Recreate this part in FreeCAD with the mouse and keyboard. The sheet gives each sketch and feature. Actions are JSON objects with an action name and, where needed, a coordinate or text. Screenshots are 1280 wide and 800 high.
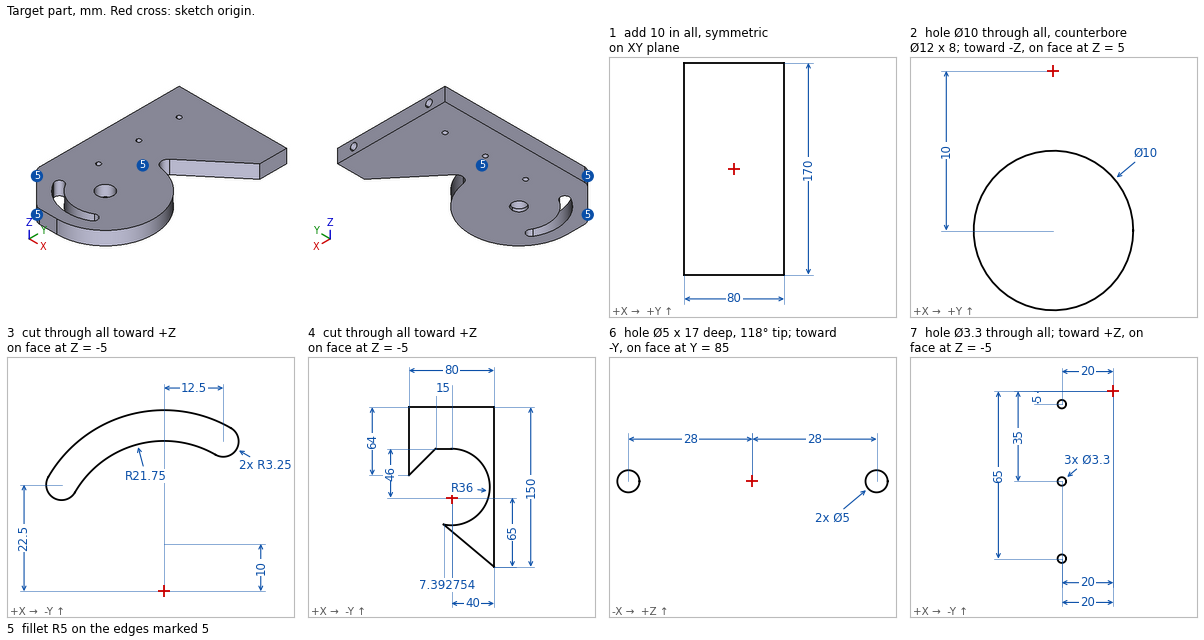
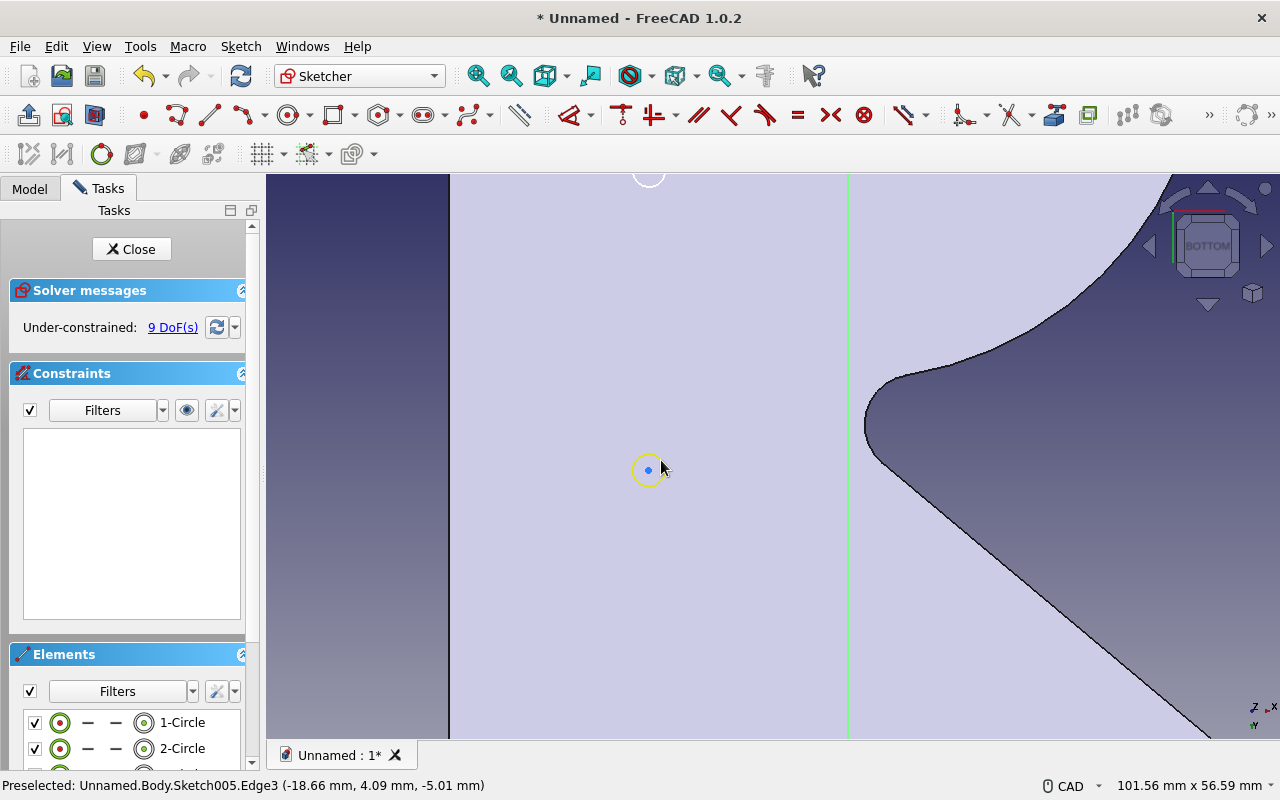
{"action": "left_click", "coordinate": [660, 459]}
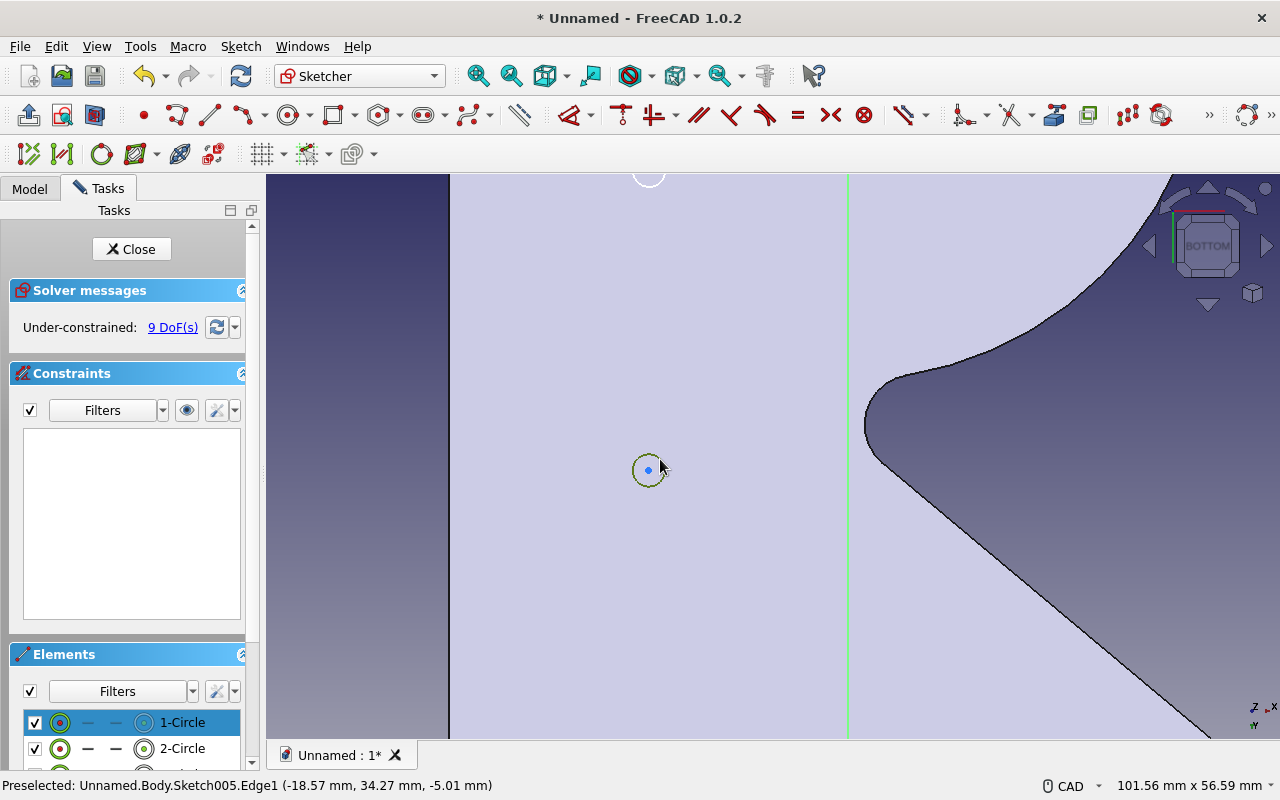
{"action": "scroll", "coordinate": [661, 460], "scroll_direction": "down", "scroll_amount": 3}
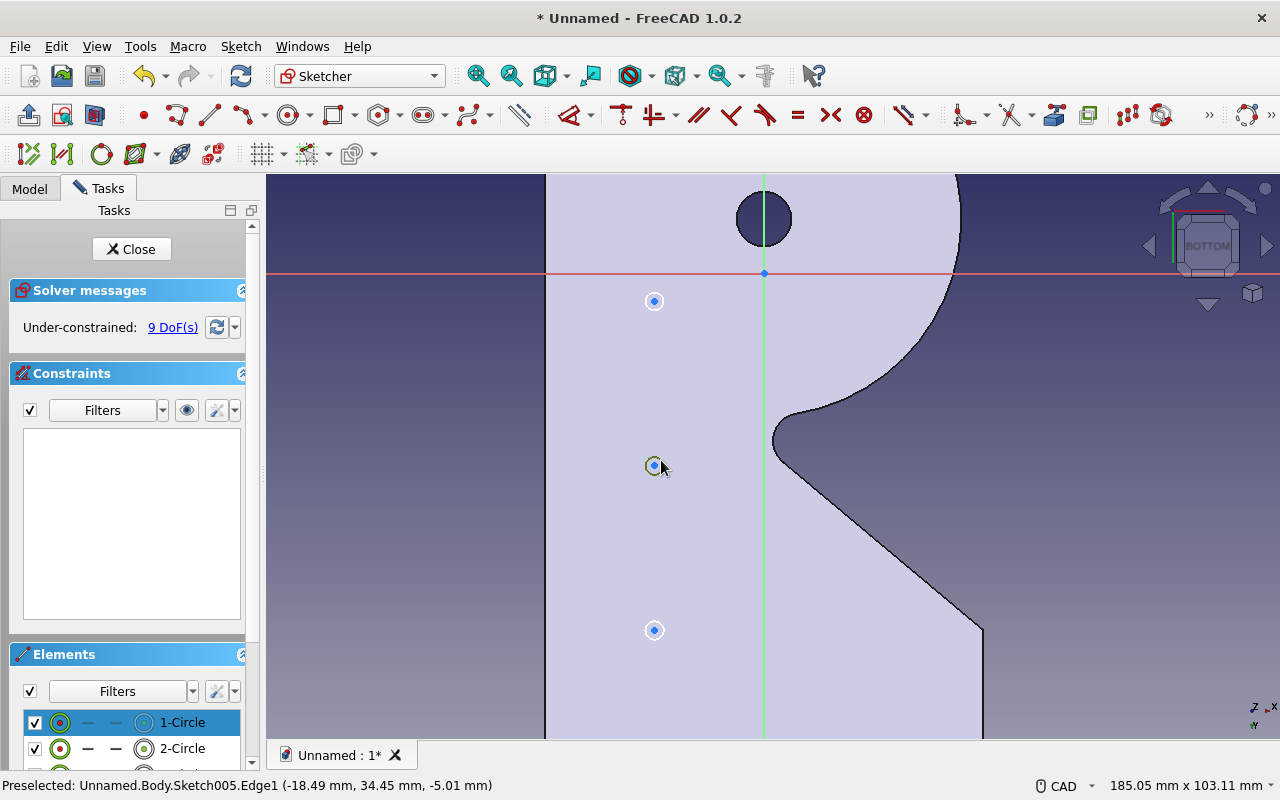
{"action": "scroll", "coordinate": [661, 624], "scroll_direction": "up", "scroll_amount": 3}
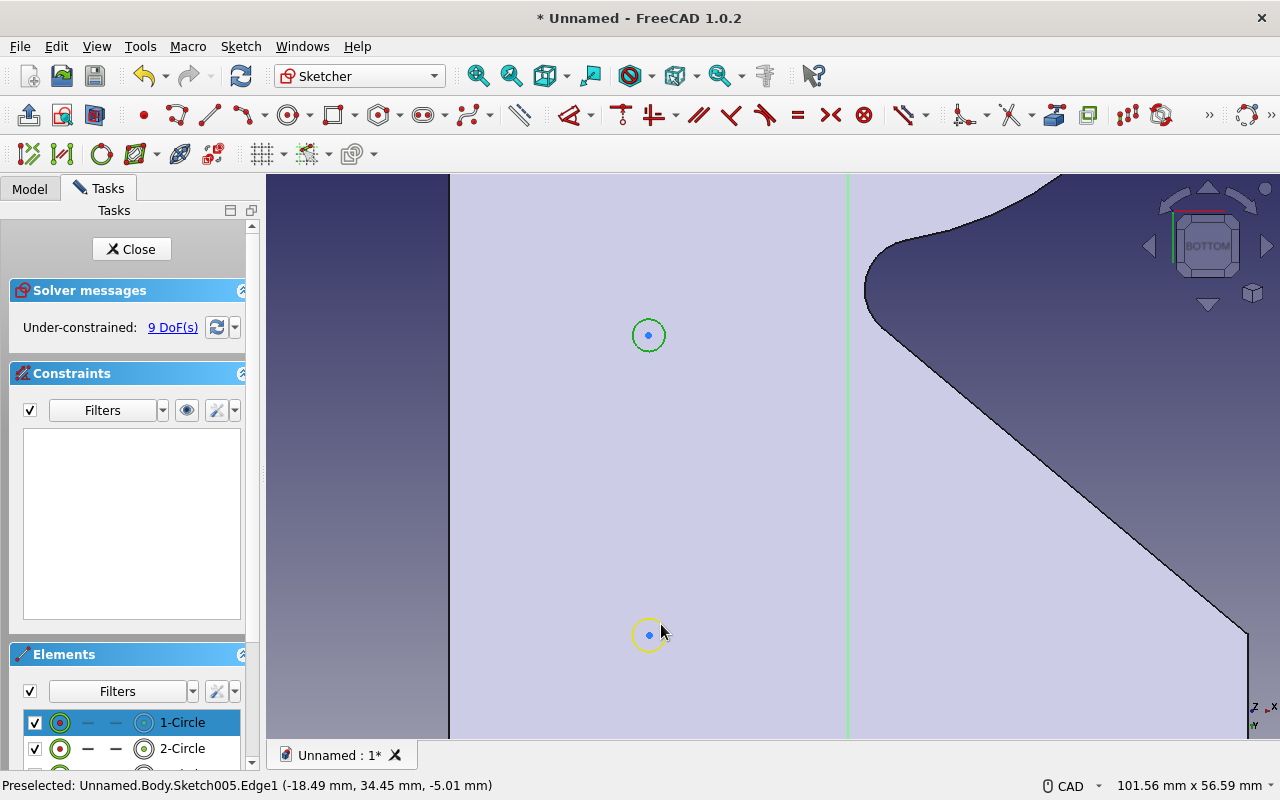
{"action": "left_click", "coordinate": [661, 623]}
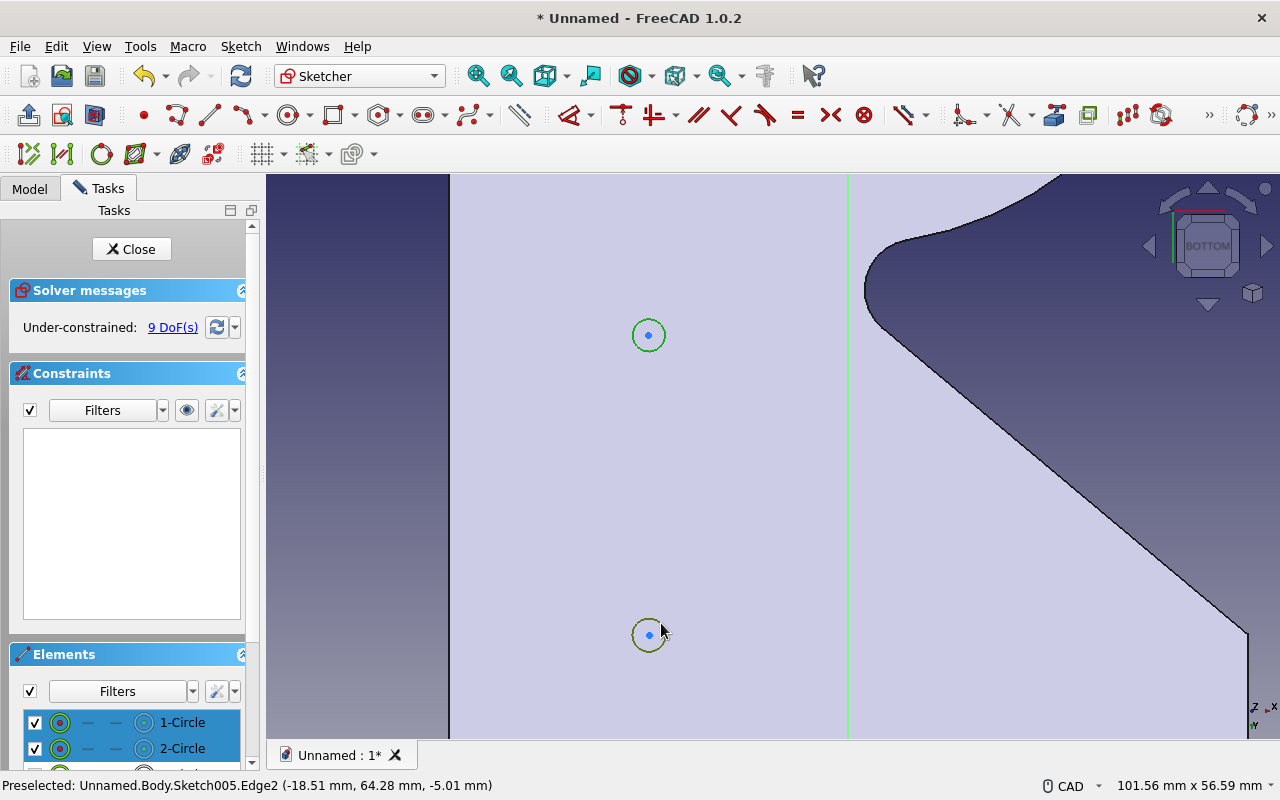
{"action": "scroll", "coordinate": [661, 625], "scroll_direction": "down", "scroll_amount": 3}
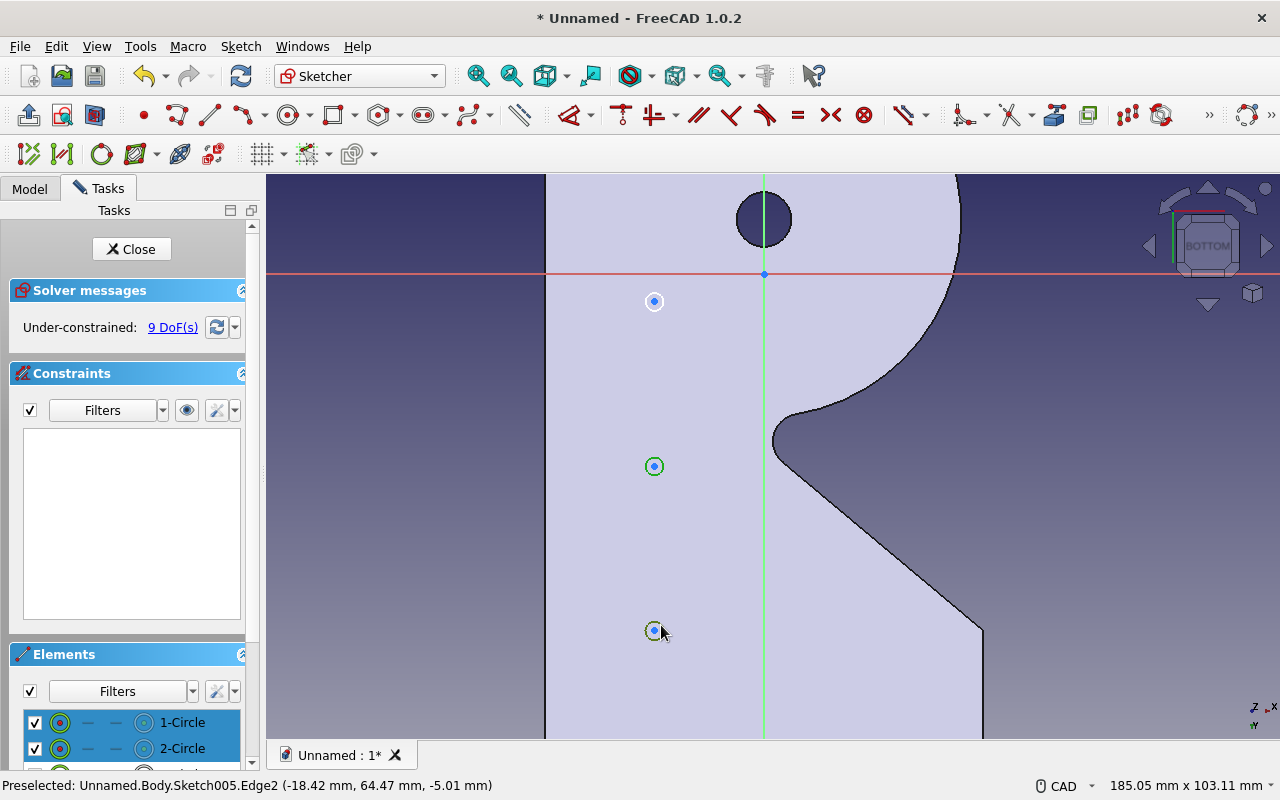
{"action": "scroll", "coordinate": [661, 296], "scroll_direction": "up", "scroll_amount": 3}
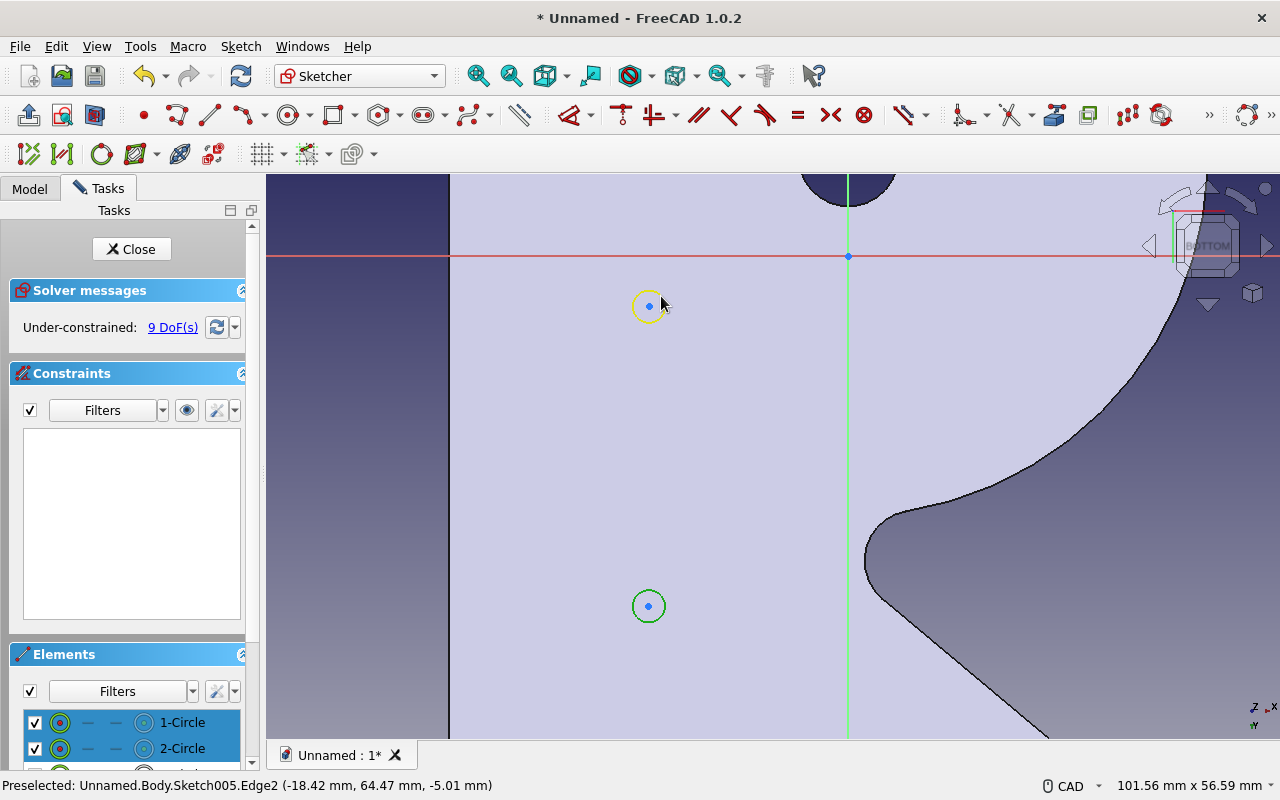
{"action": "left_click", "coordinate": [660, 295]}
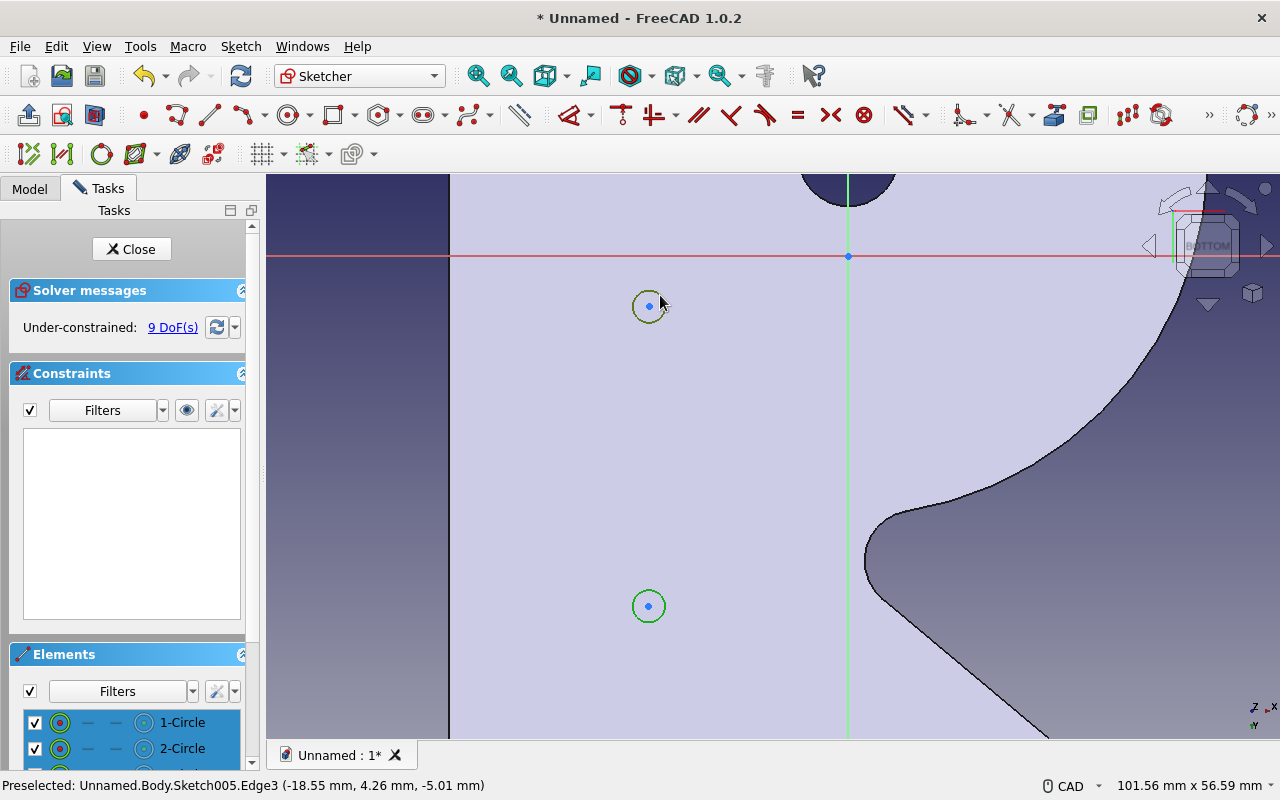
{"action": "key", "text": "e"}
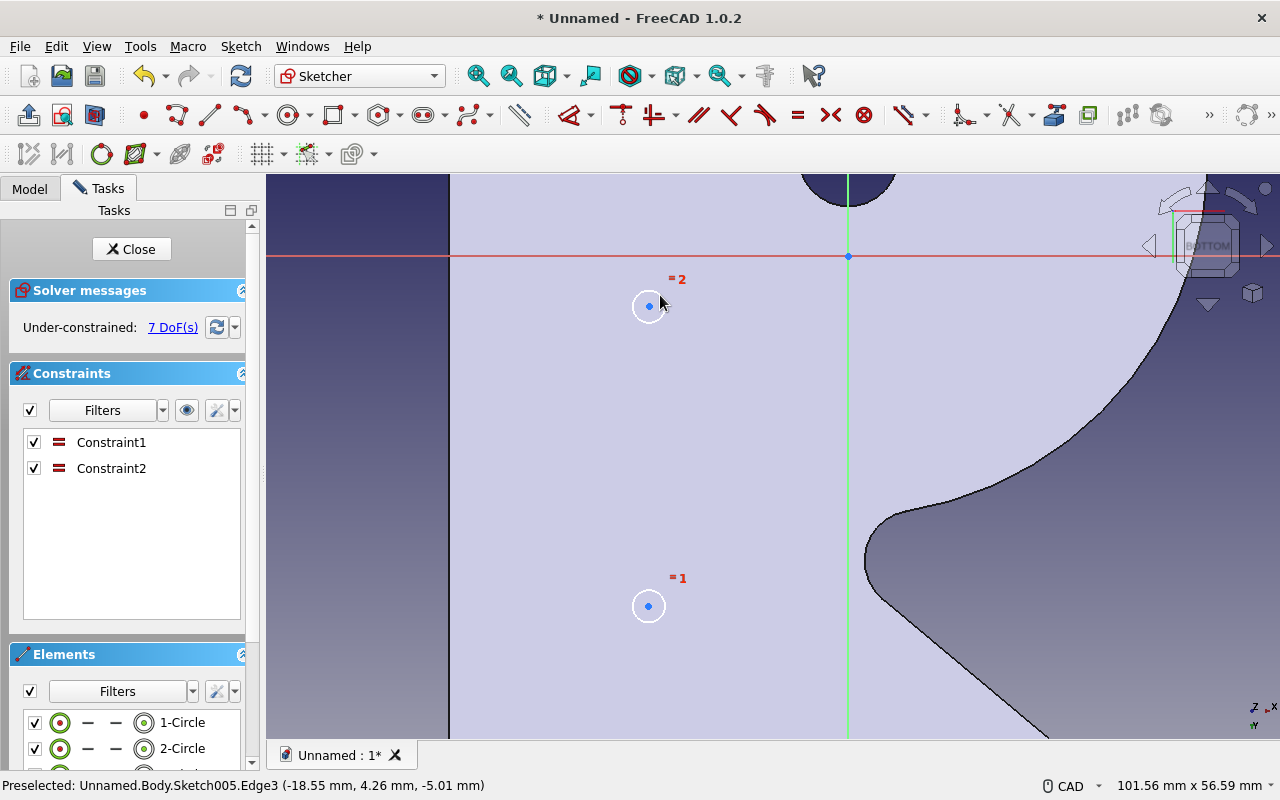
{"action": "key", "text": "d"}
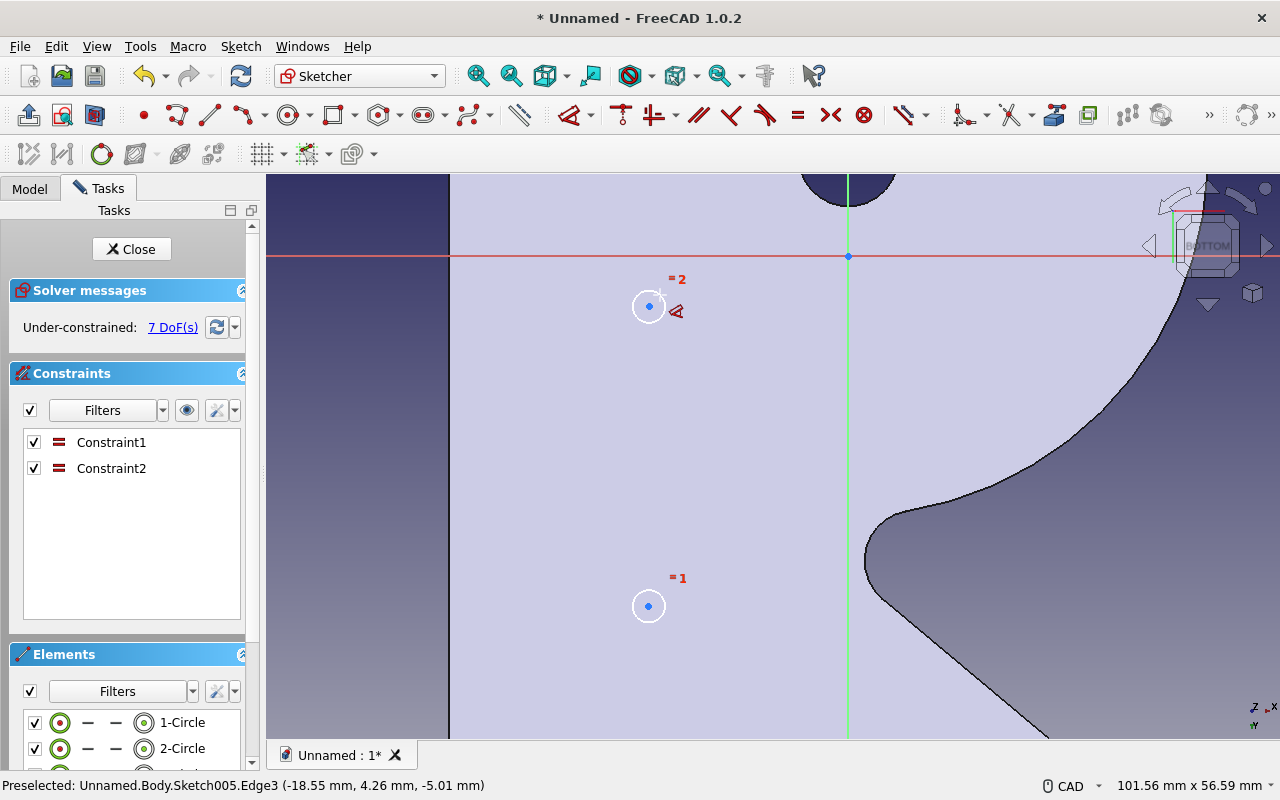
{"action": "left_click", "coordinate": [660, 595]}
{"action": "left_click", "coordinate": [682, 572]}